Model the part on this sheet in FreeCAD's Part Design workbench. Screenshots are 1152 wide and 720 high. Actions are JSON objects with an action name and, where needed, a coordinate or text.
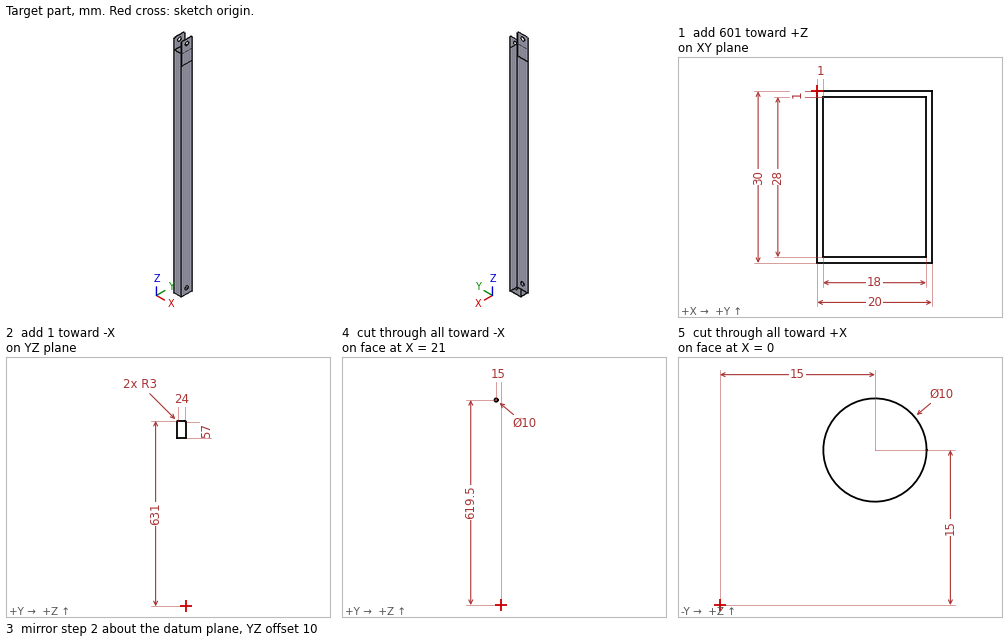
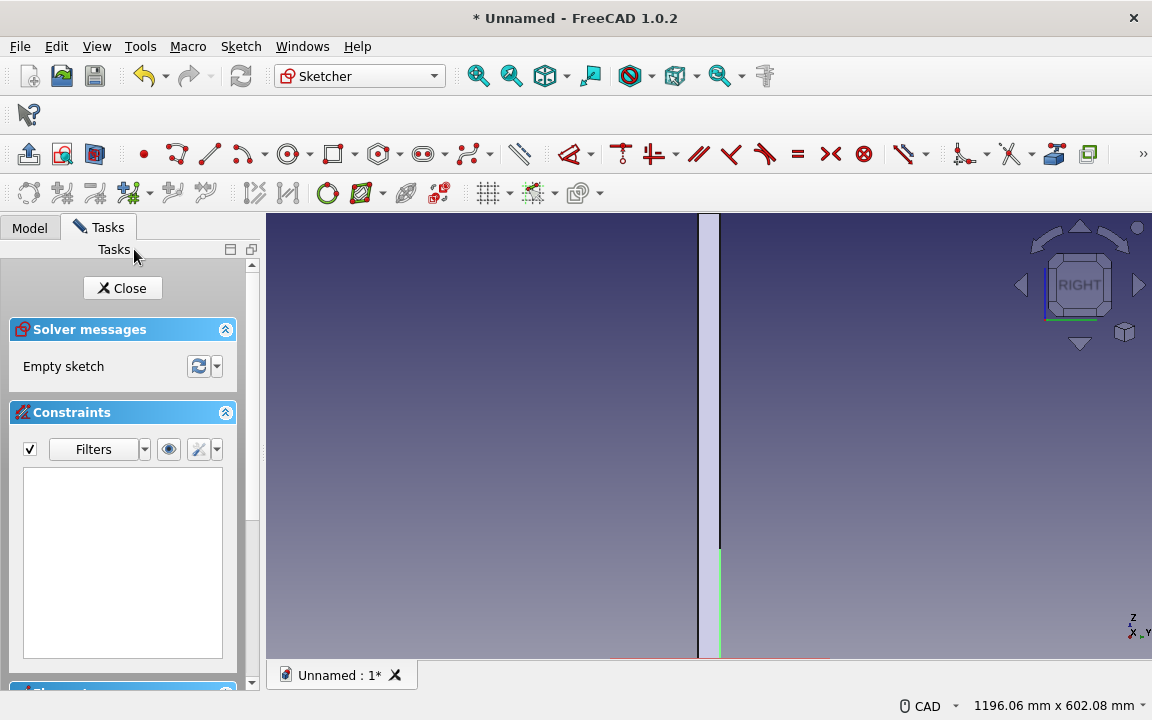
{"action": "scroll", "coordinate": [640, 436], "scroll_direction": "down", "scroll_amount": 5}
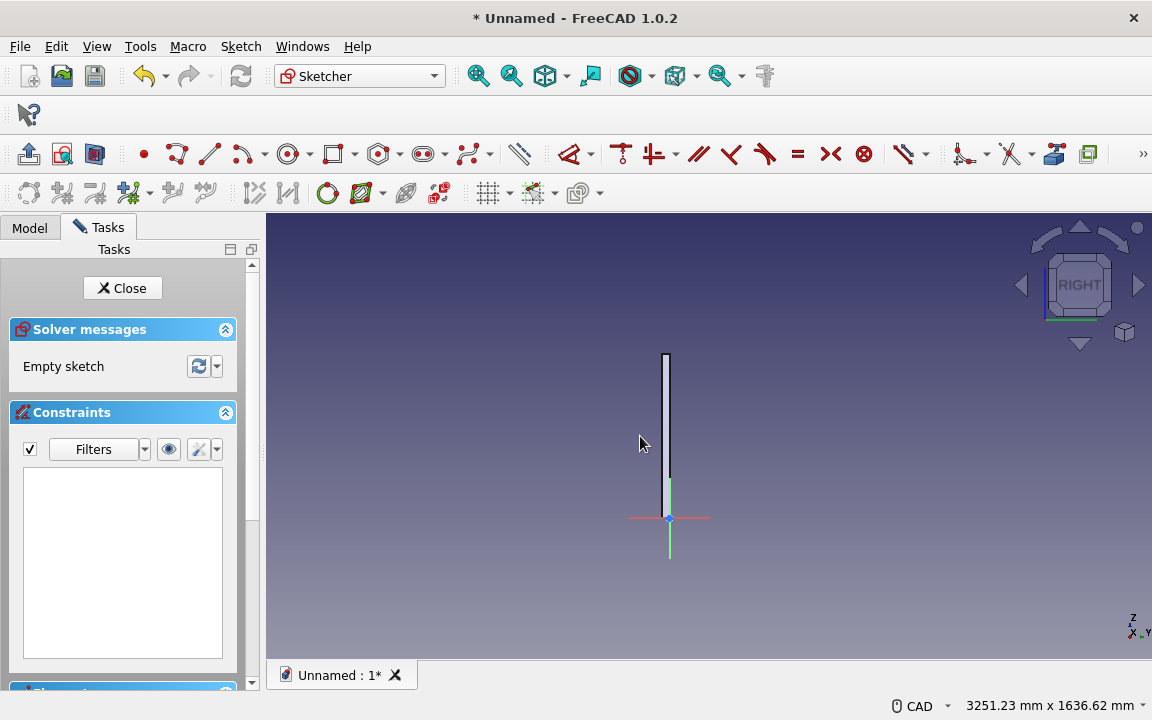
{"action": "scroll", "coordinate": [667, 349], "scroll_direction": "up", "scroll_amount": 14}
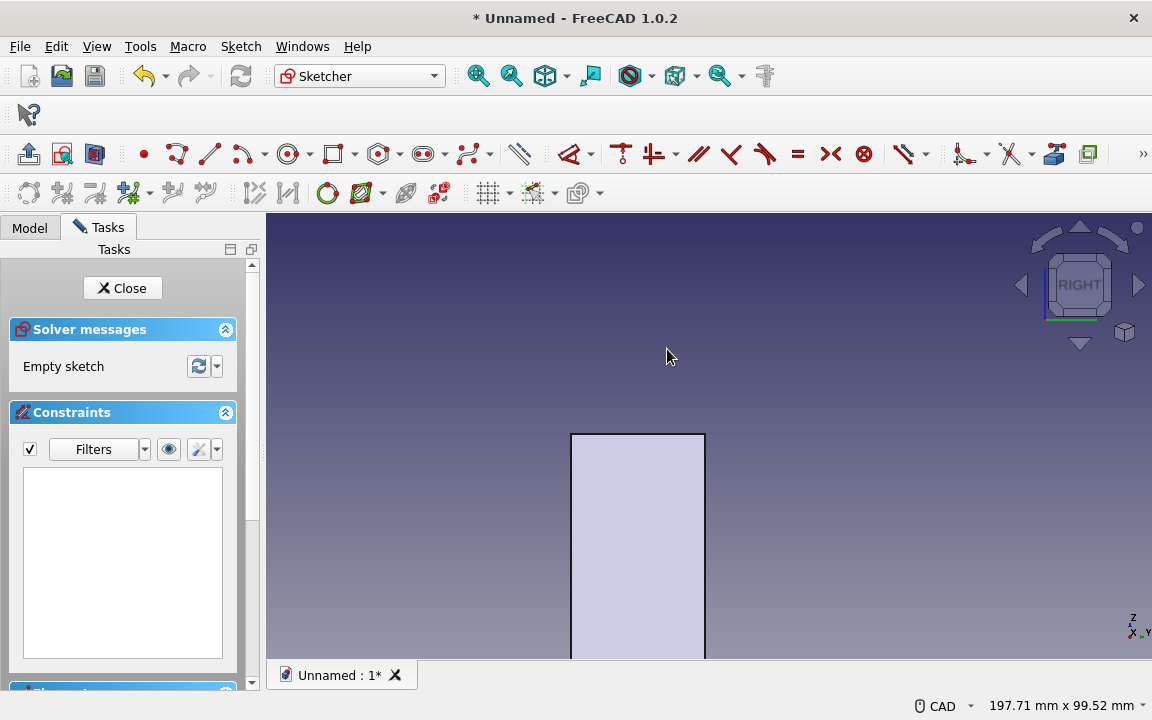
{"action": "key", "text": "g l"}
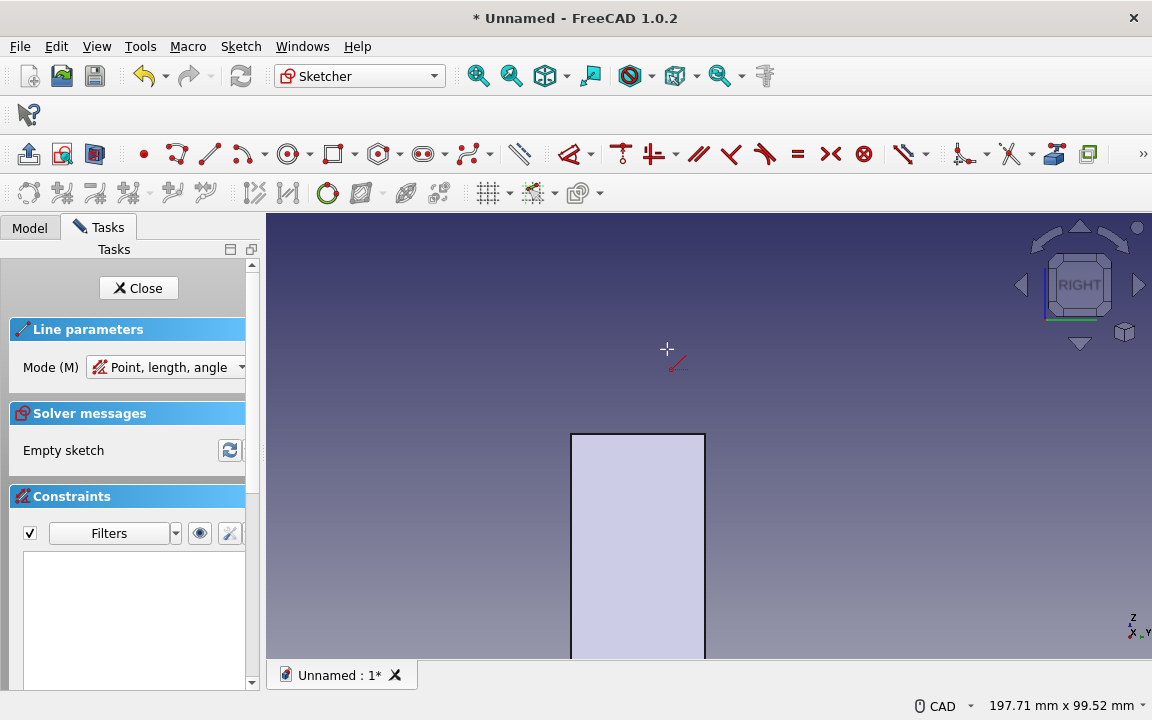
{"action": "left_click", "coordinate": [584, 299]}
{"action": "left_click", "coordinate": [692, 299]}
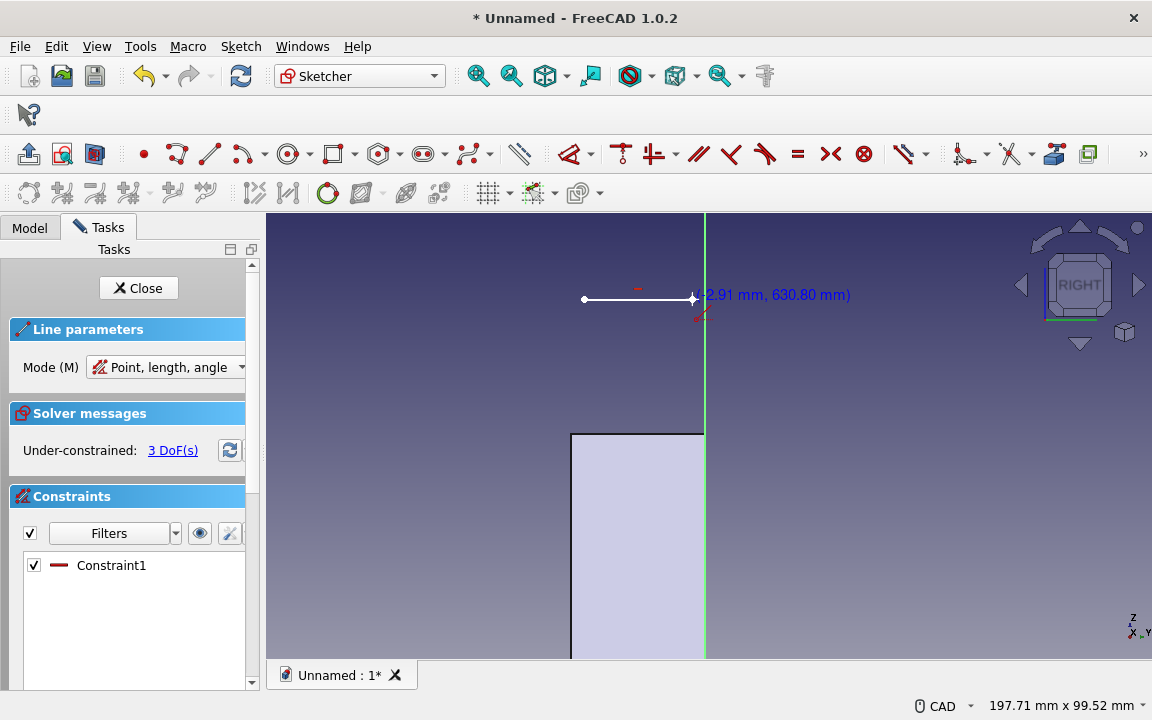
{"action": "left_click", "coordinate": [177, 154]}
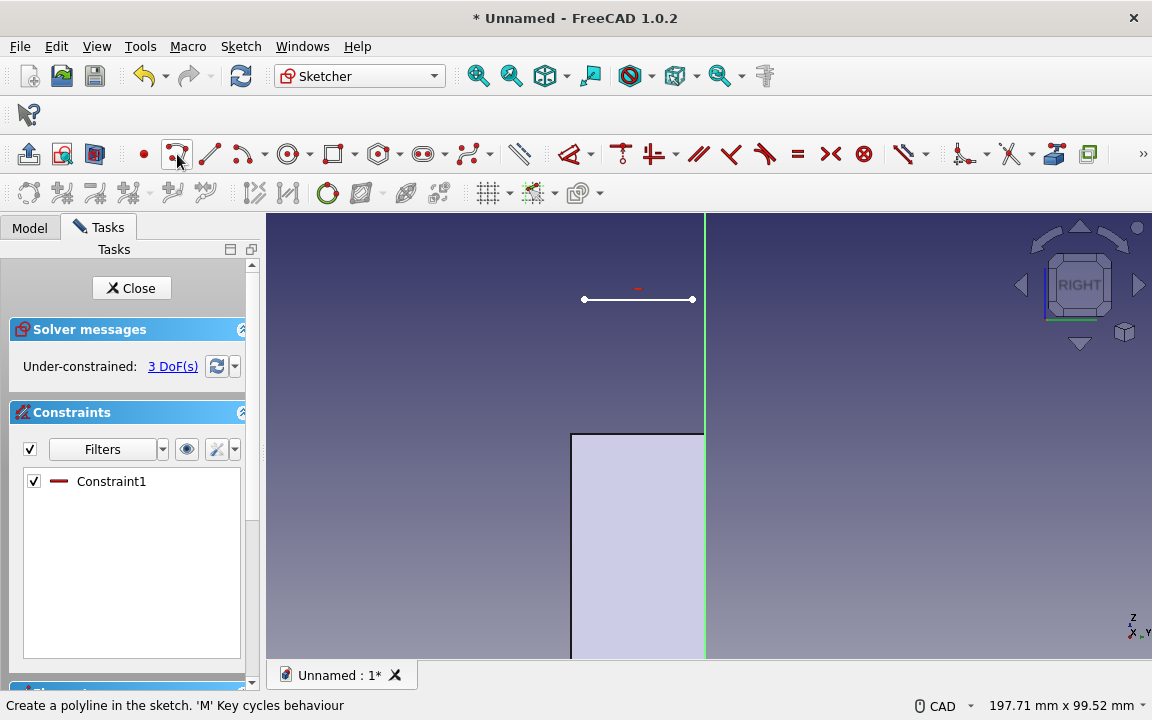
{"action": "left_click", "coordinate": [705, 313]}
{"action": "left_click", "coordinate": [696, 568]}
{"action": "left_click", "coordinate": [571, 568]}
{"action": "left_click", "coordinate": [571, 313]}
{"action": "right_click", "coordinate": [571, 313]}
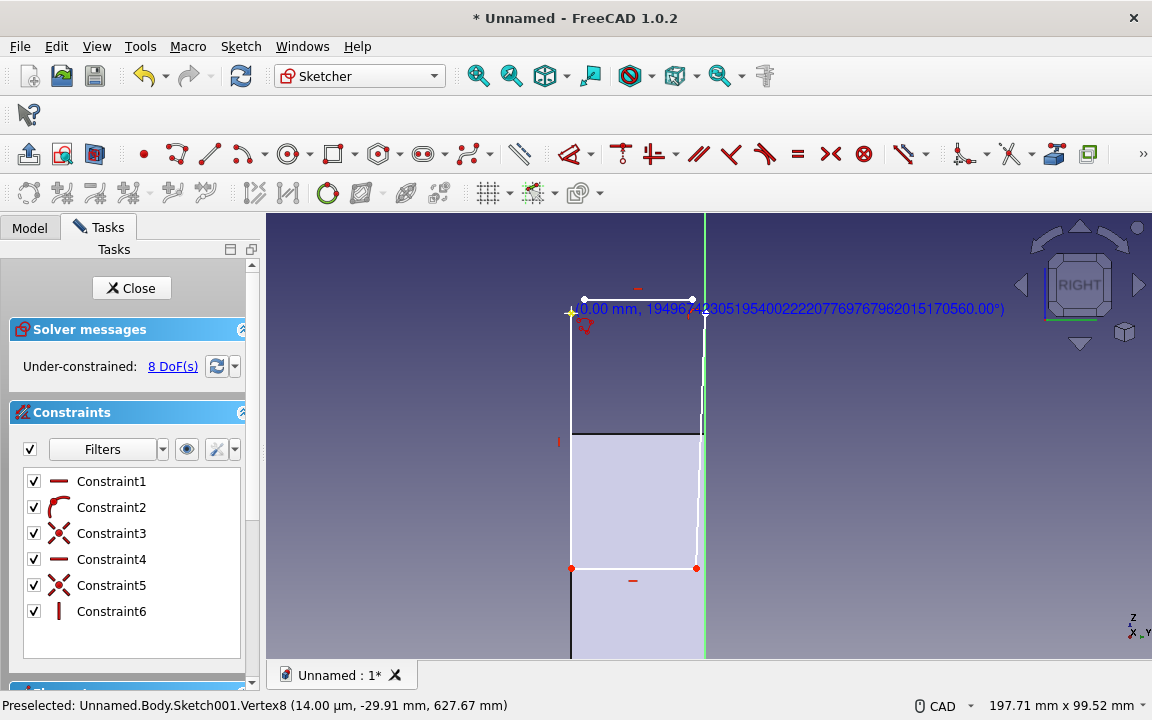
{"action": "key", "text": "g 3 a"}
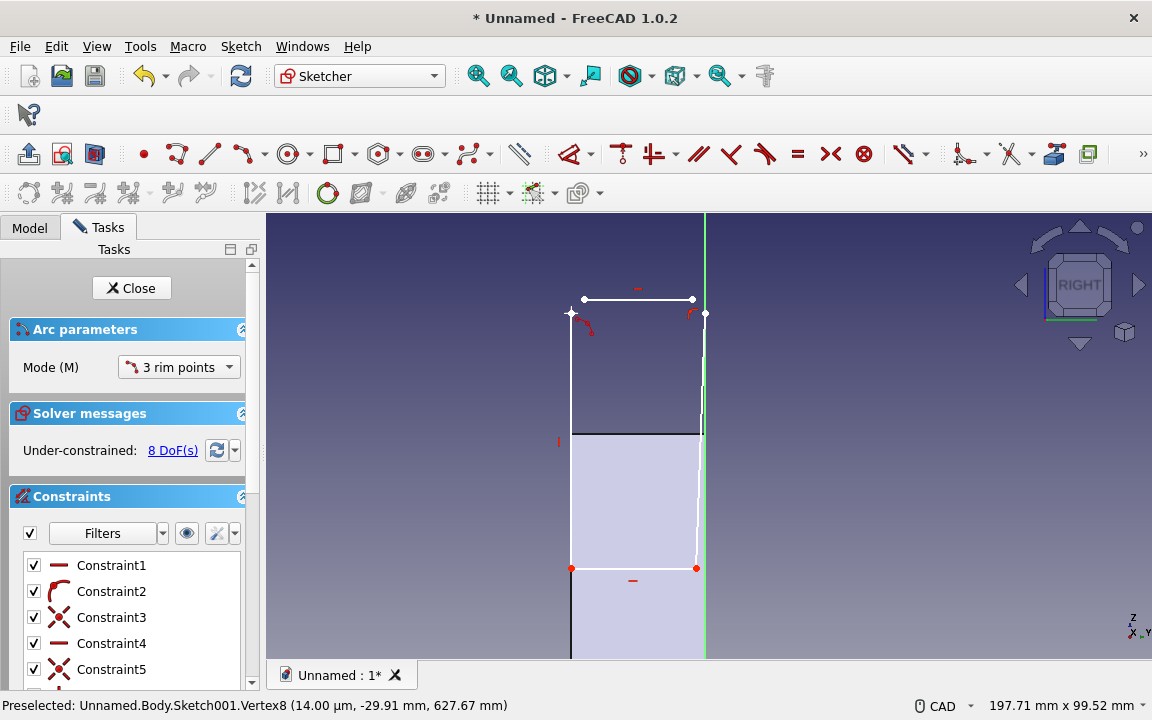
{"action": "left_click", "coordinate": [692, 300]}
{"action": "left_click", "coordinate": [705, 314]}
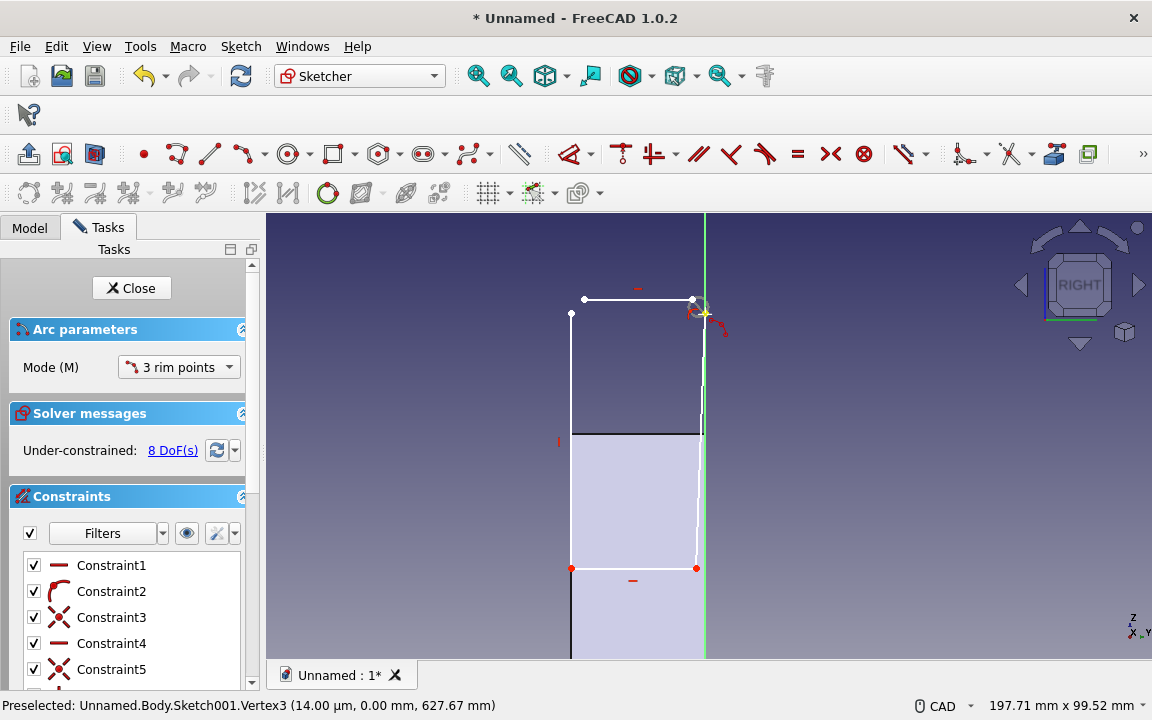
{"action": "scroll", "coordinate": [701, 303], "scroll_direction": "up", "scroll_amount": 7}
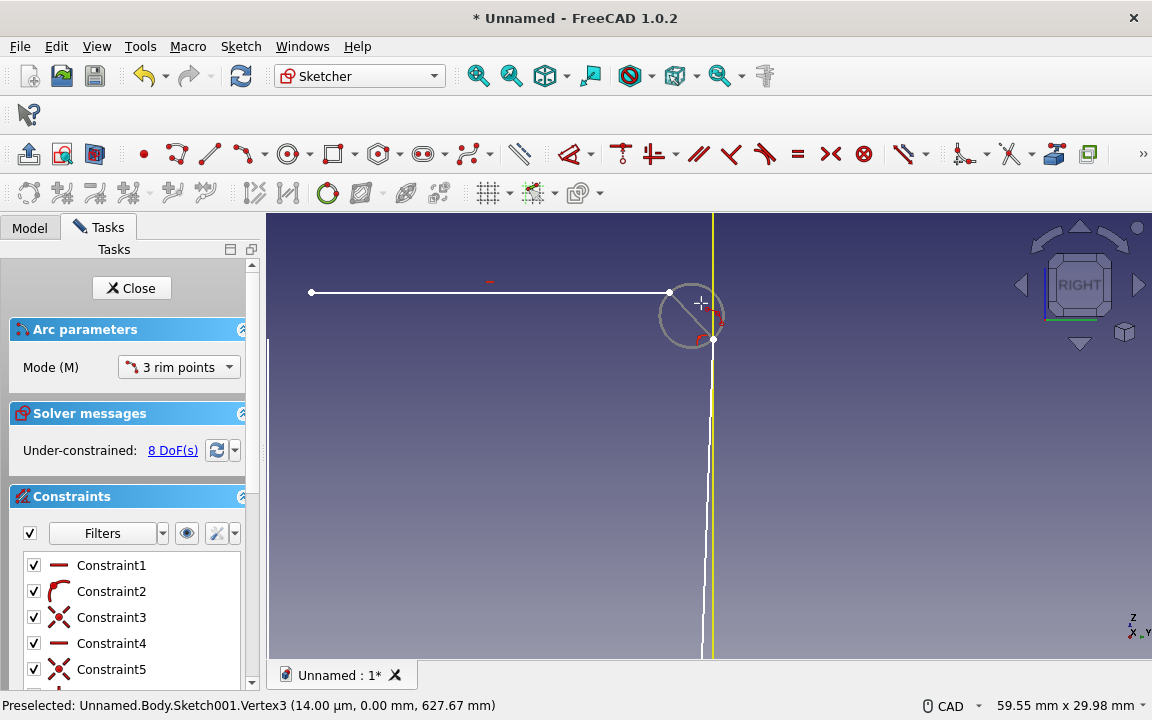
{"action": "left_click", "coordinate": [700, 302]}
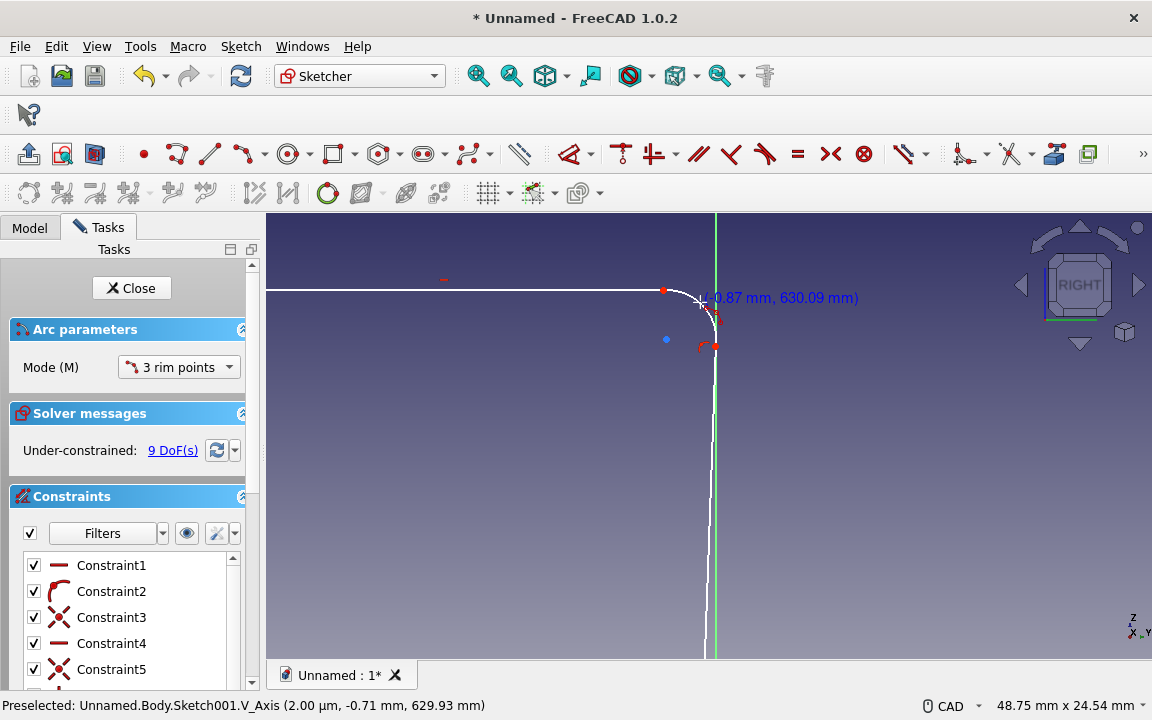
{"action": "scroll", "coordinate": [705, 306], "scroll_direction": "down", "scroll_amount": 7}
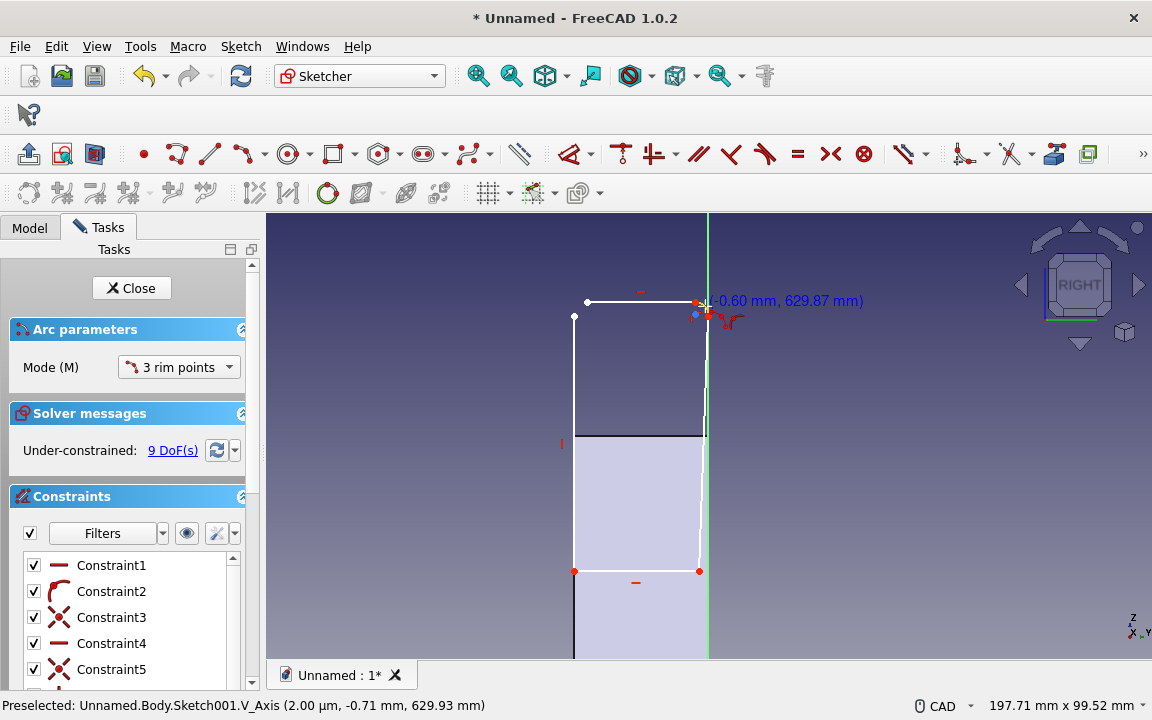
{"action": "left_click", "coordinate": [574, 316]}
{"action": "left_click", "coordinate": [587, 302]}